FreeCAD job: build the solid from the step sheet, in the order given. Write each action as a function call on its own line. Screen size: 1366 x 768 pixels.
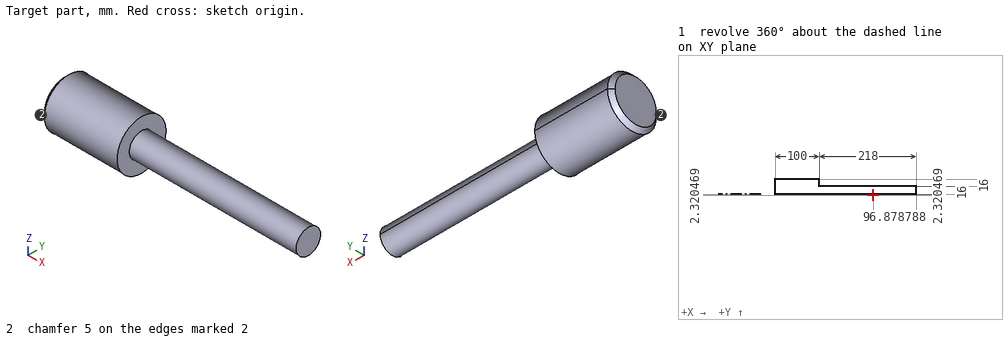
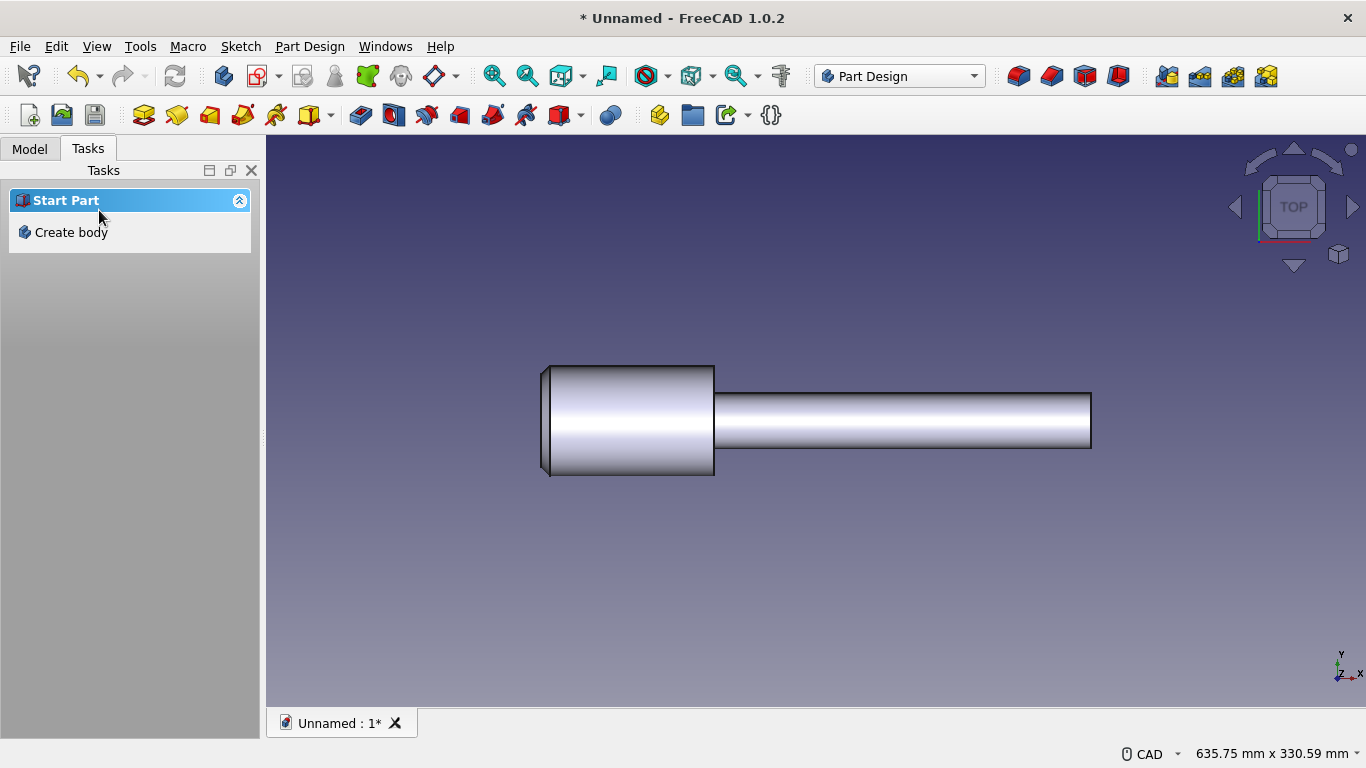
key(0)